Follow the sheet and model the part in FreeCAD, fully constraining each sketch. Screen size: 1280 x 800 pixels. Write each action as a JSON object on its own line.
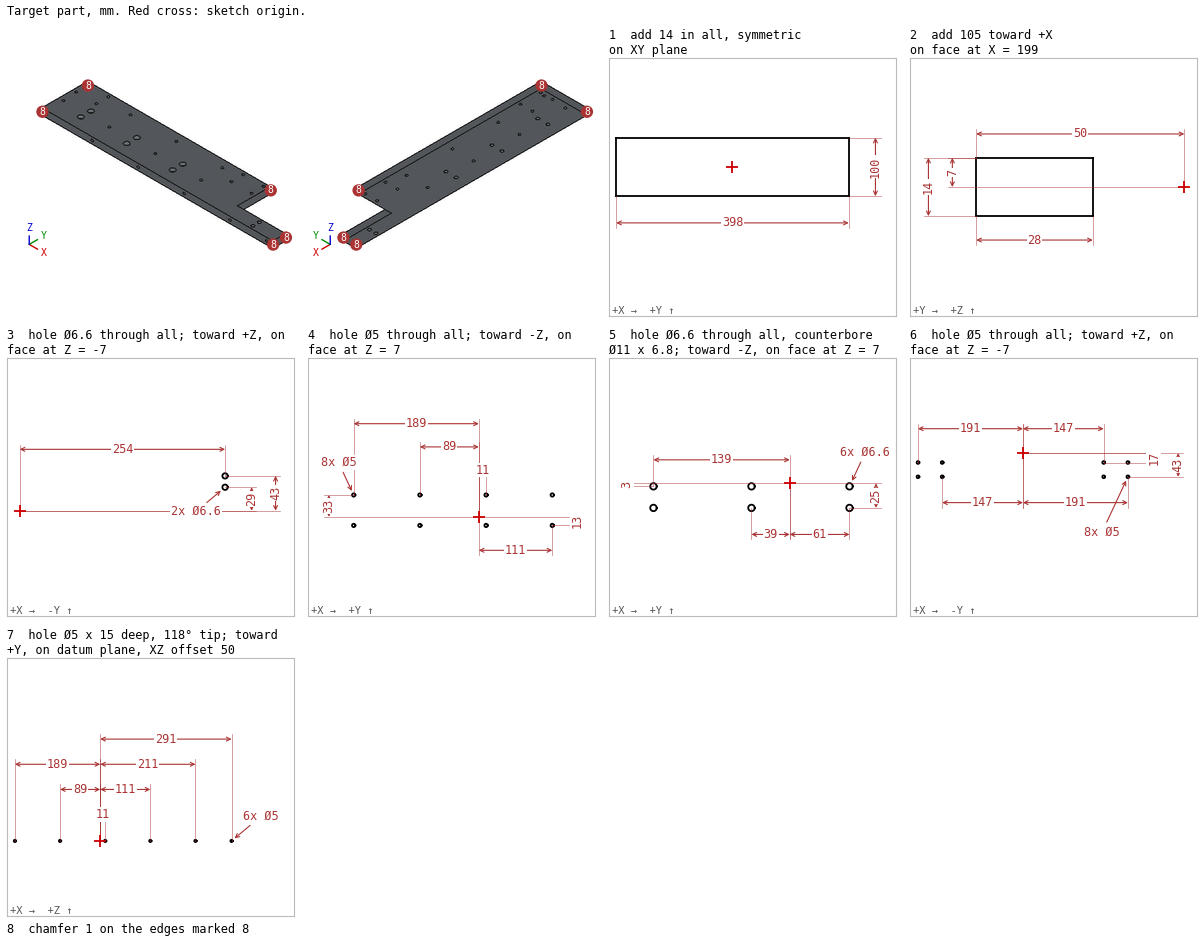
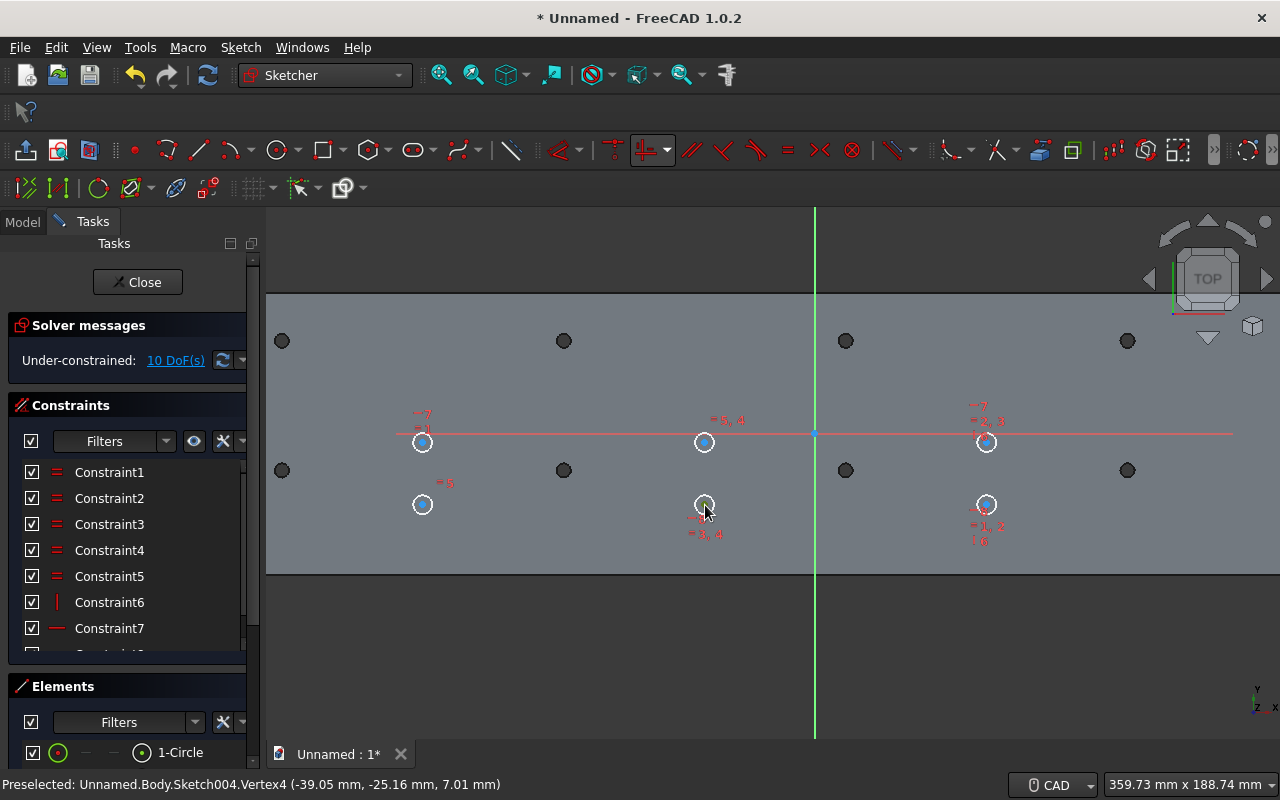
{"action": "left_click", "coordinate": [705, 443]}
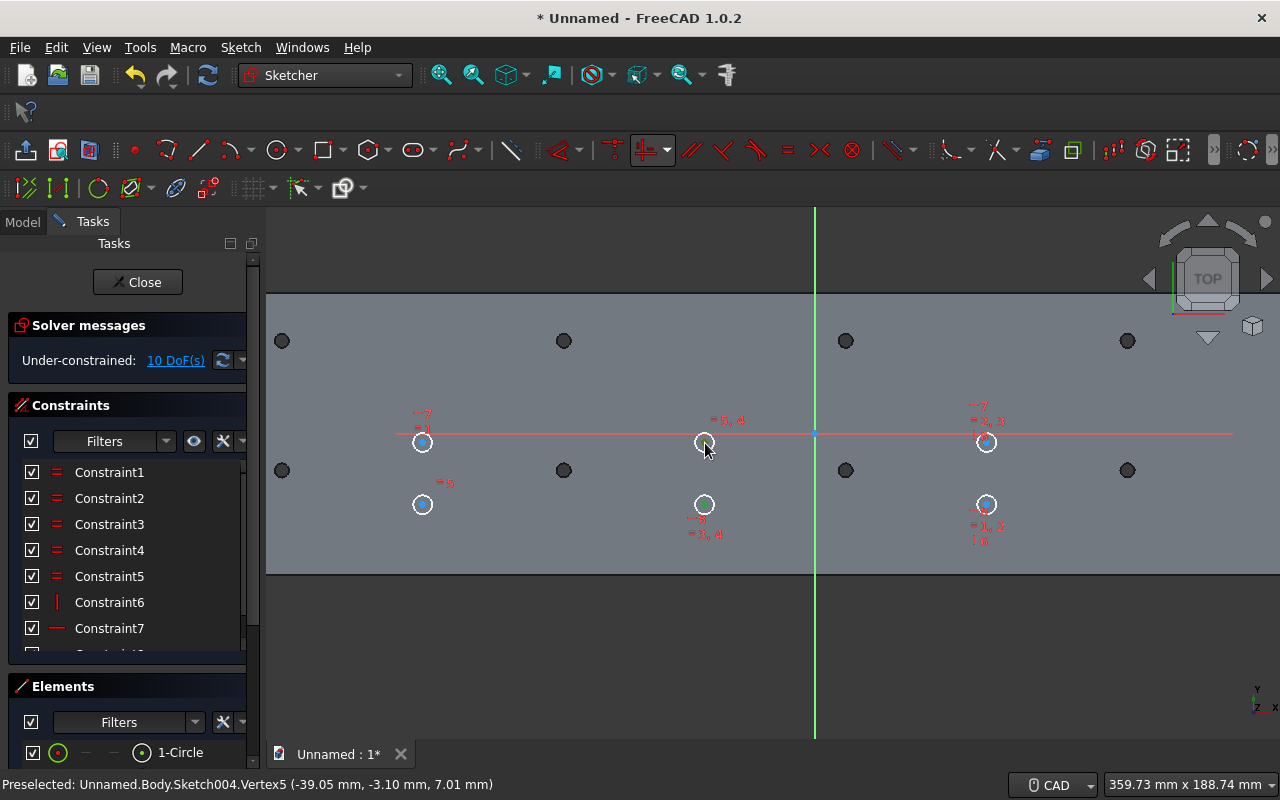
{"action": "key", "text": "v"}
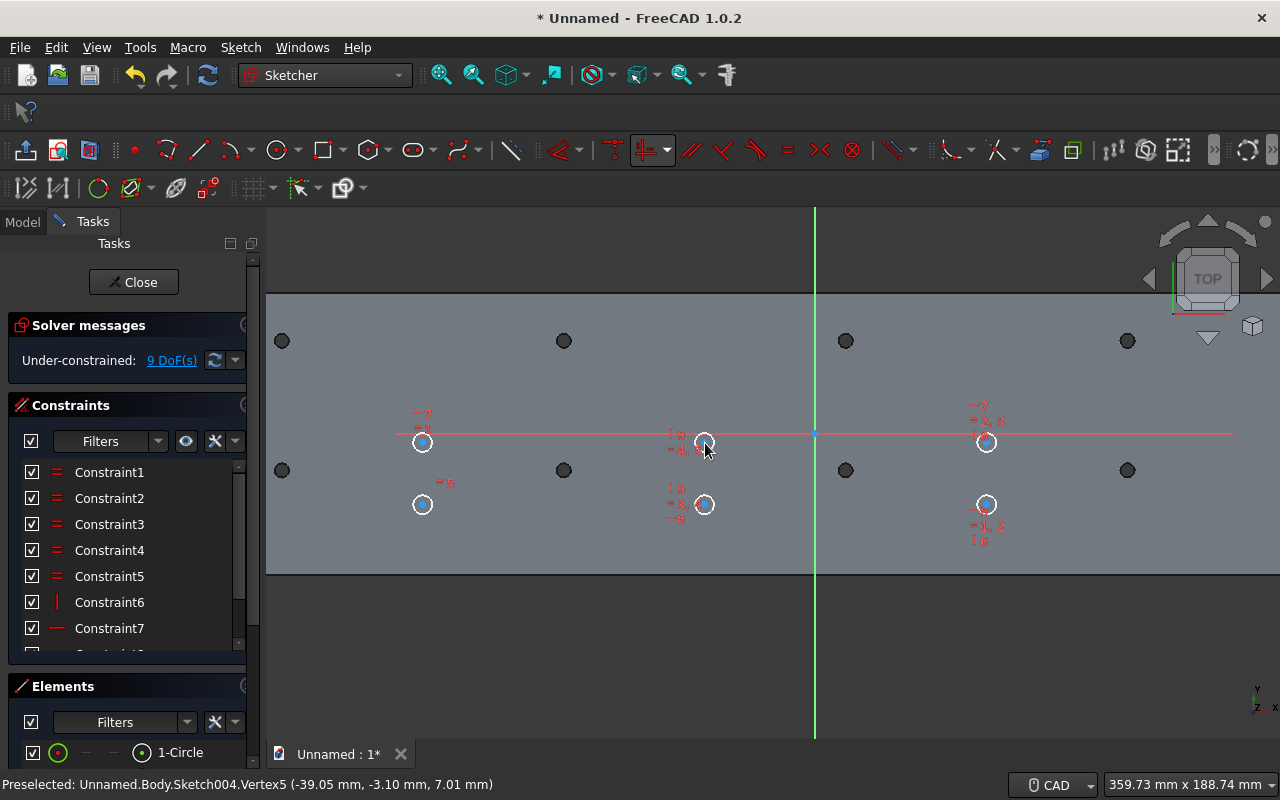
{"action": "left_click", "coordinate": [423, 443]}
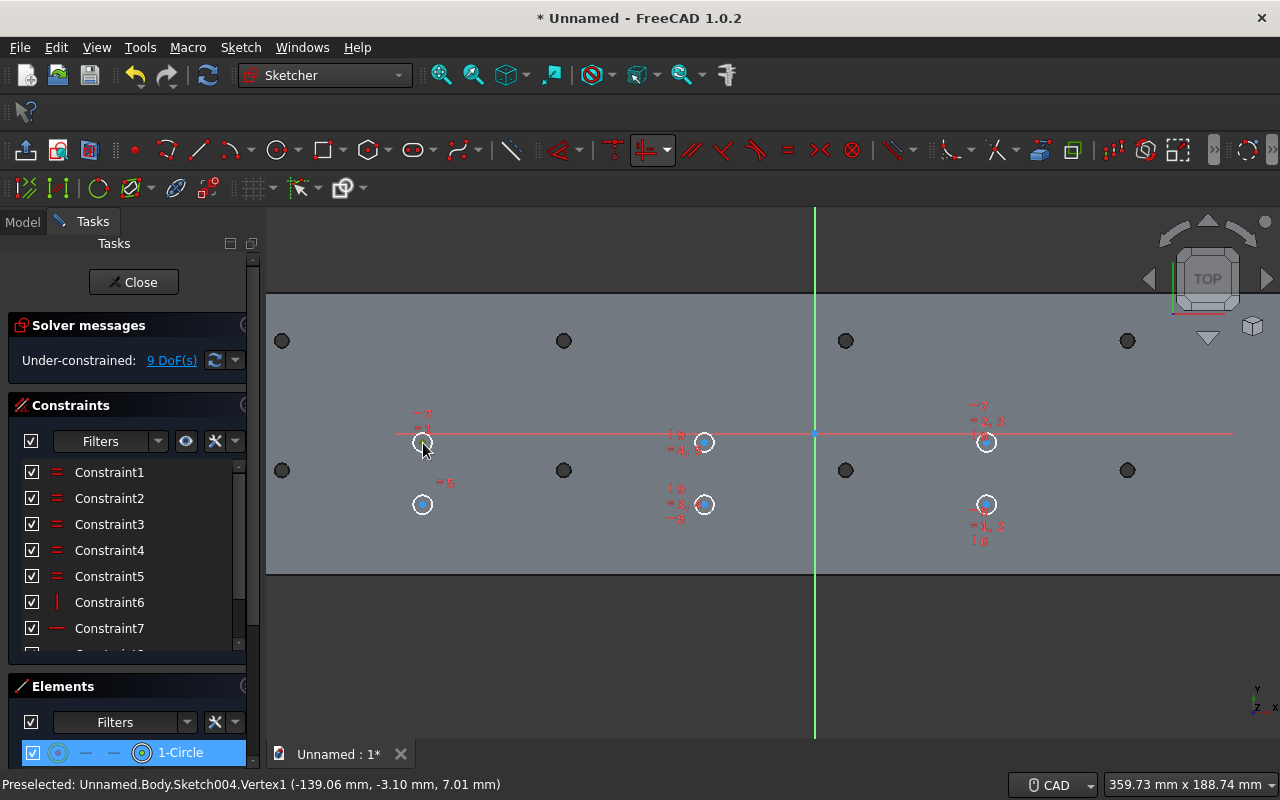
{"action": "left_click", "coordinate": [705, 443]}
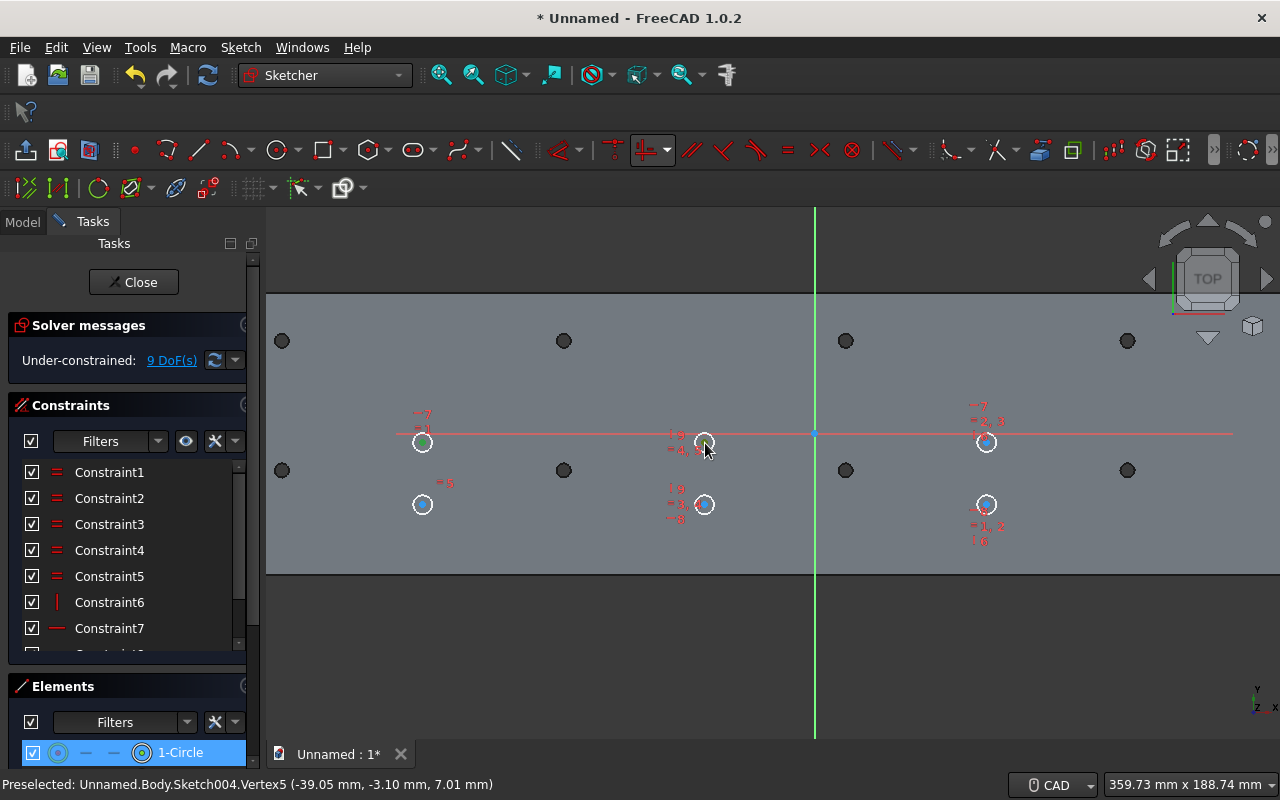
{"action": "key", "text": "h"}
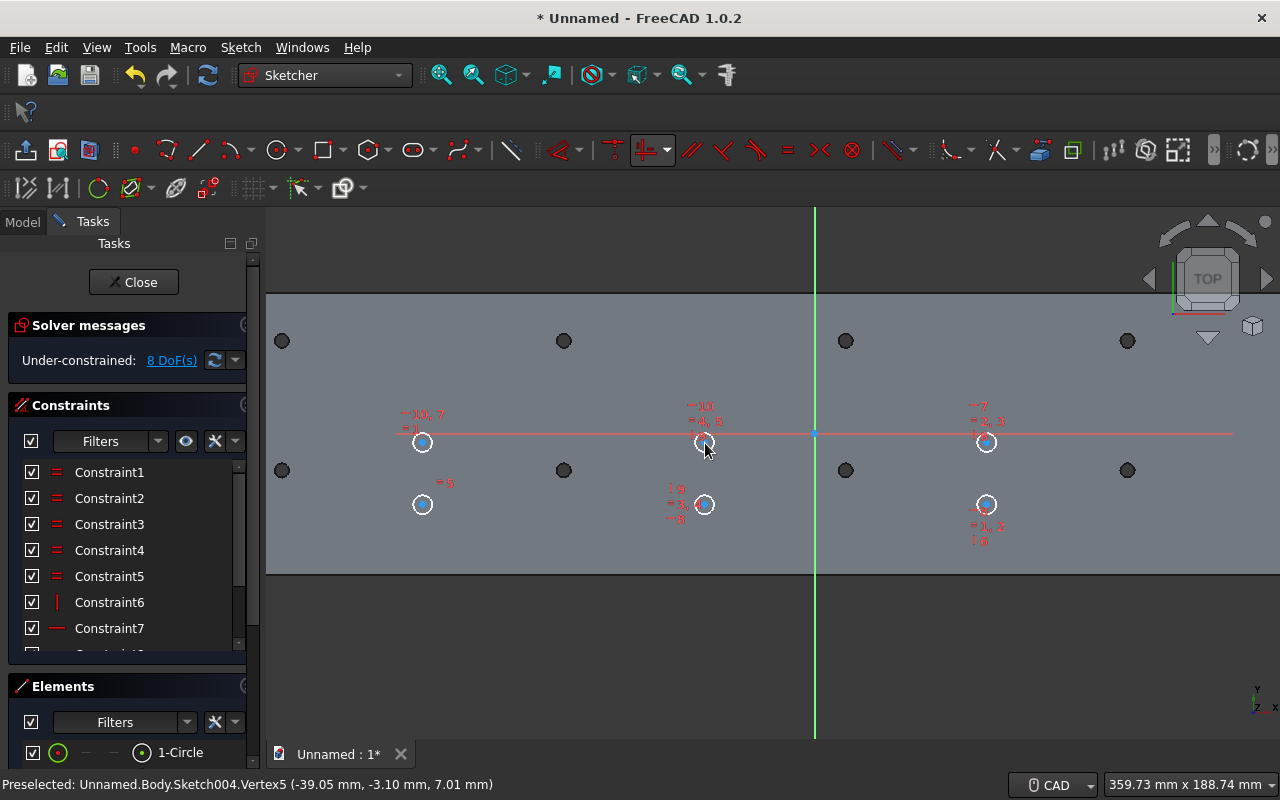
{"action": "left_click", "coordinate": [423, 443]}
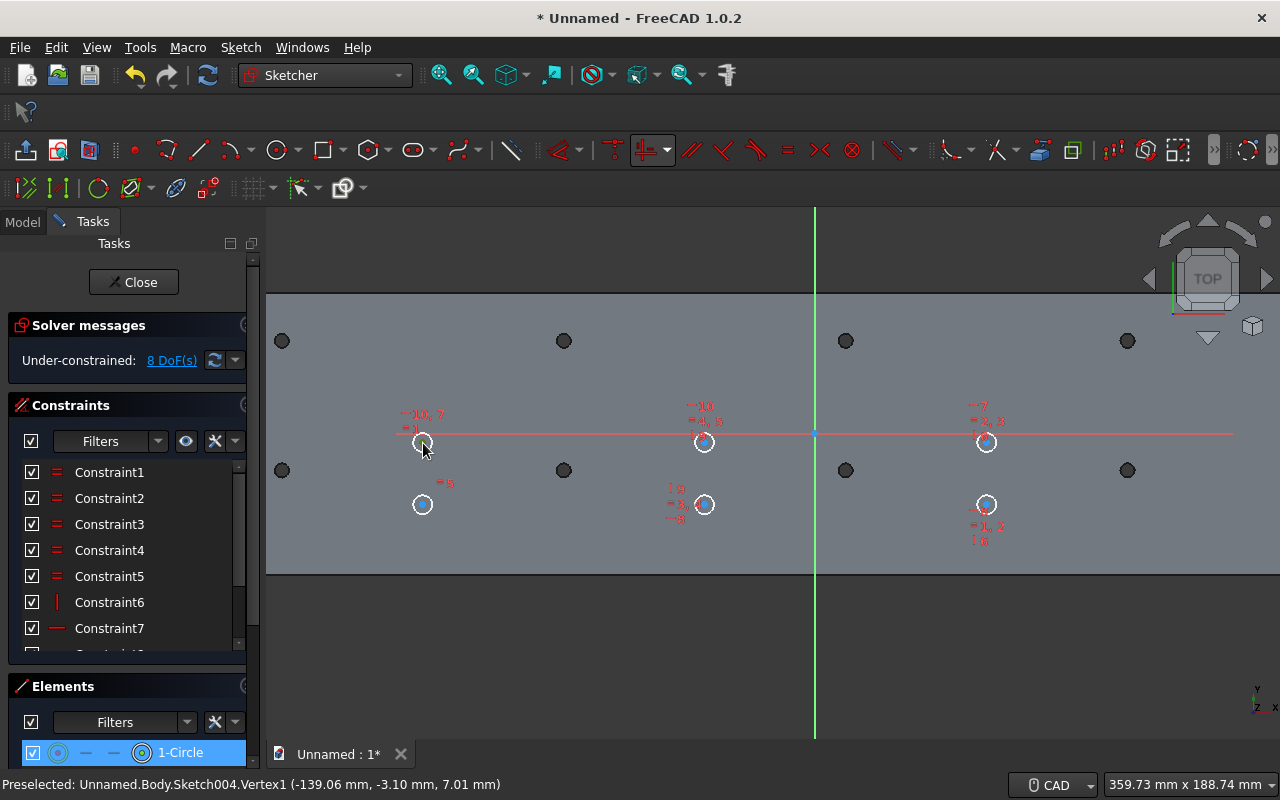
{"action": "left_click", "coordinate": [423, 505]}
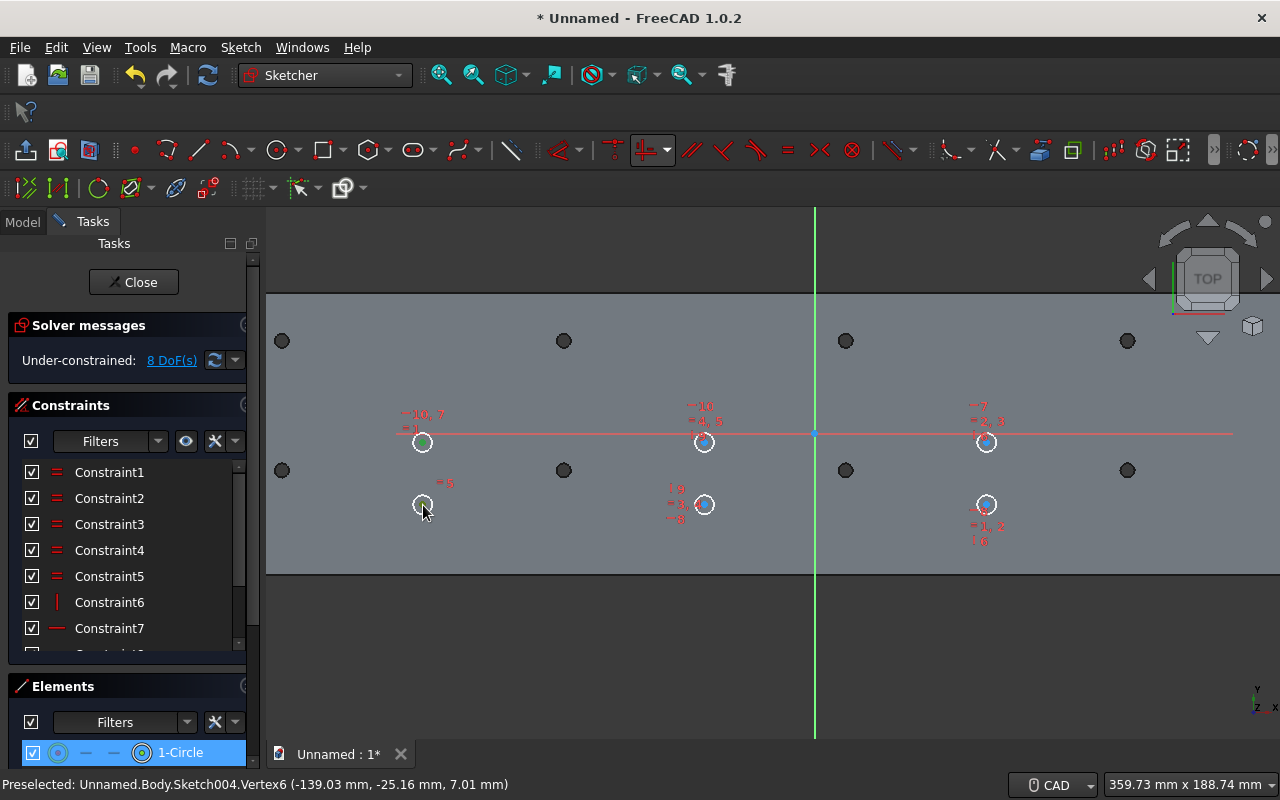
{"action": "key", "text": "v"}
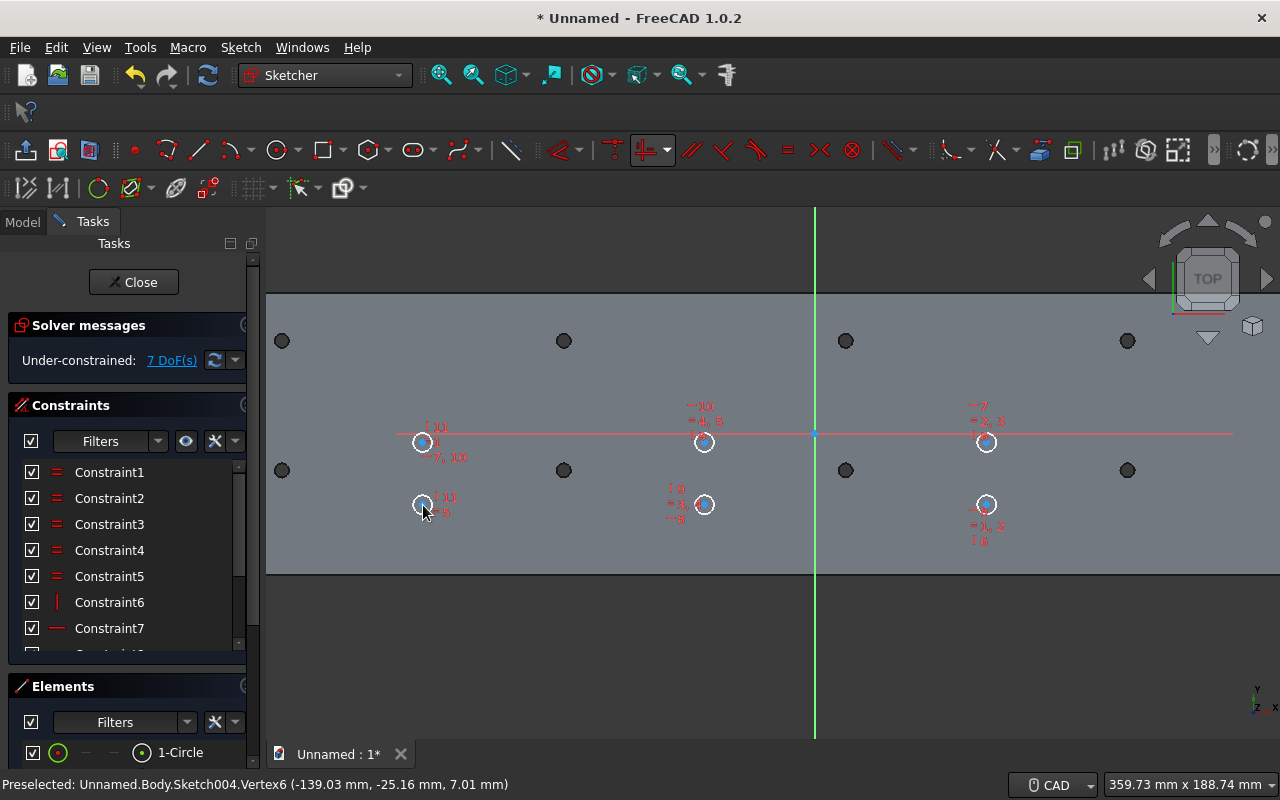
{"action": "left_click", "coordinate": [705, 505]}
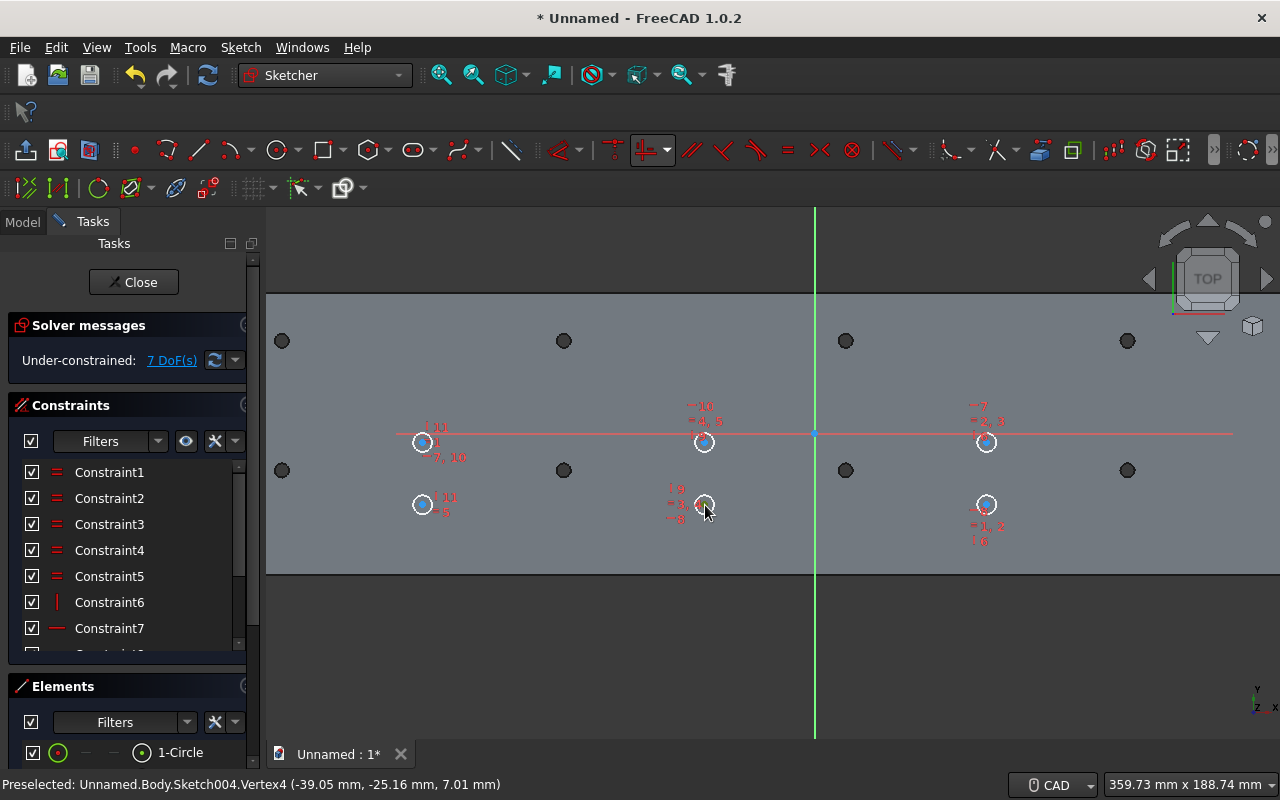
{"action": "left_click", "coordinate": [423, 505]}